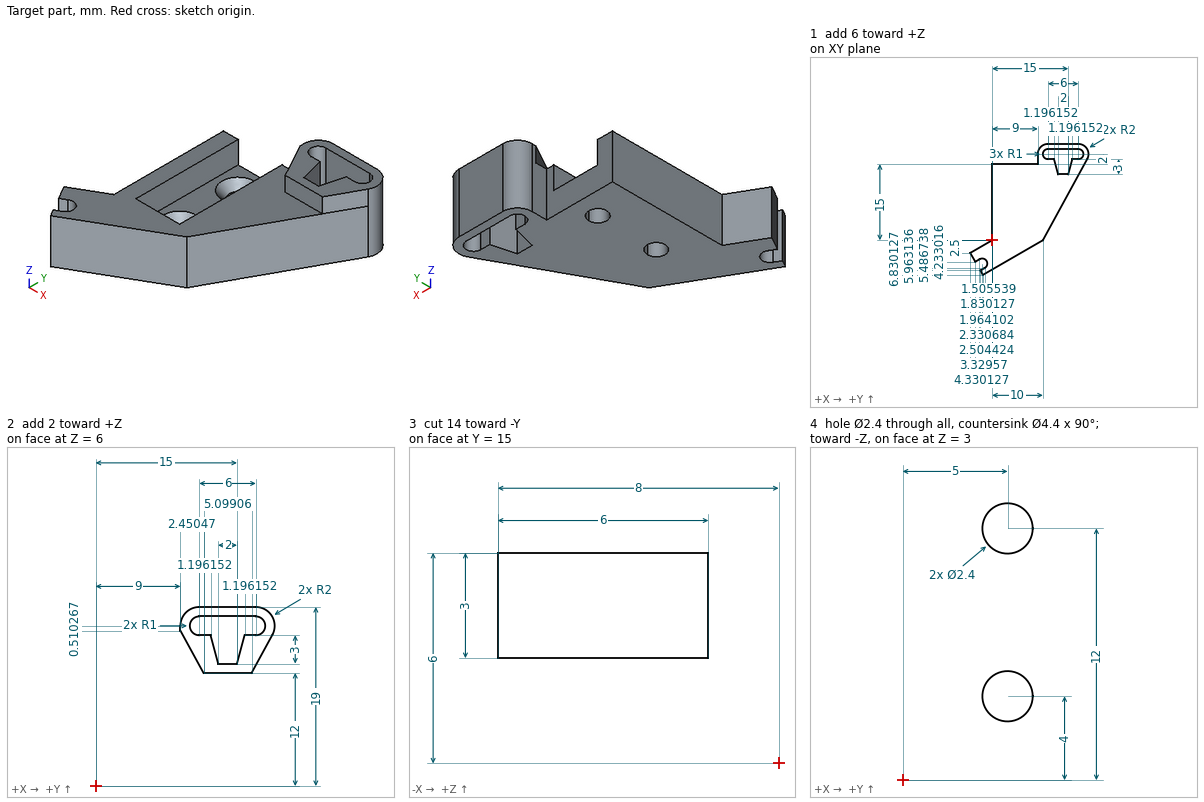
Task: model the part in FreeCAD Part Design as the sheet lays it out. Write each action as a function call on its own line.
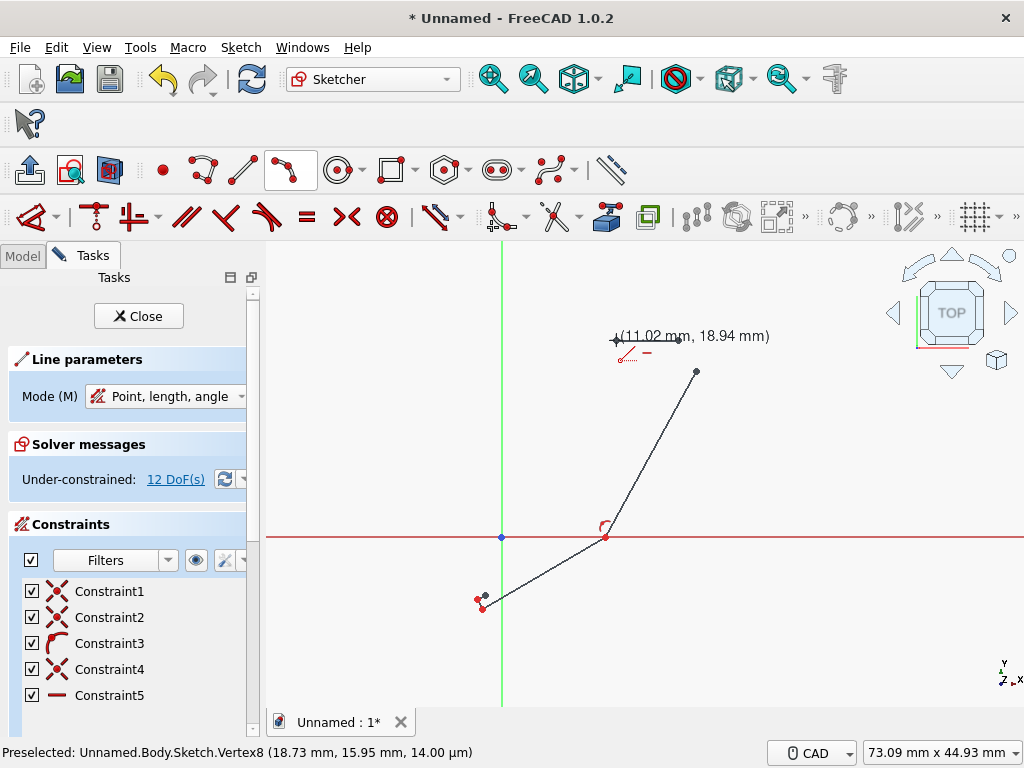
click(204, 170)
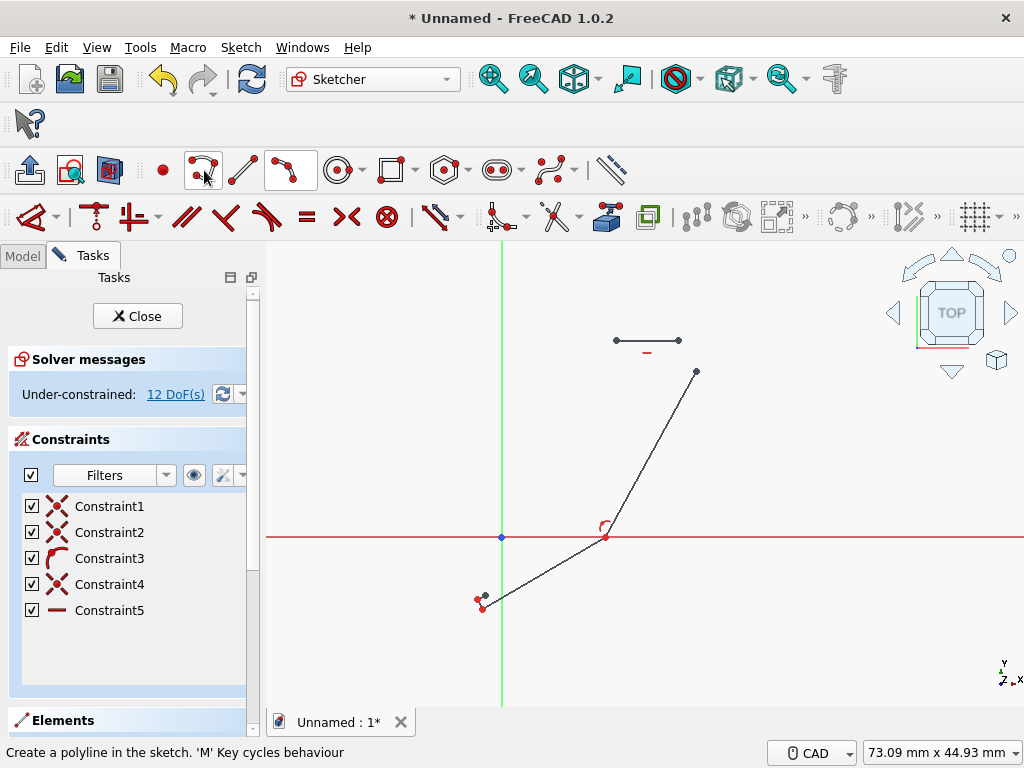
click(595, 361)
click(595, 382)
click(502, 382)
click(502, 537)
click(457, 563)
click(467, 581)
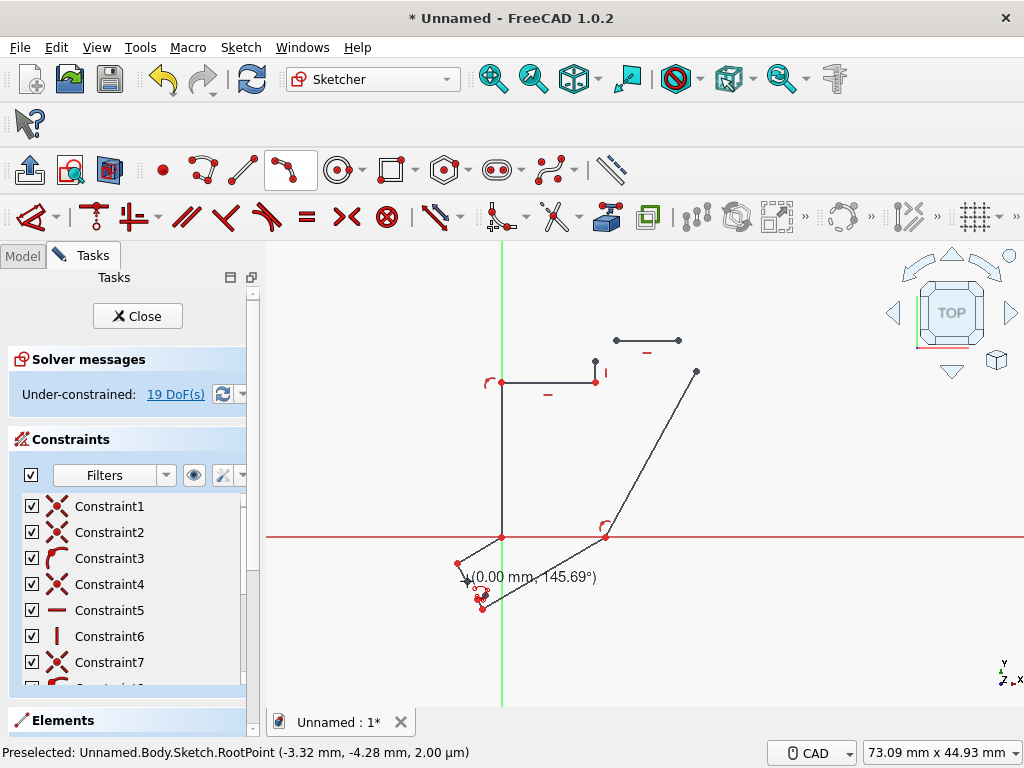
scroll(476, 576, up, 3)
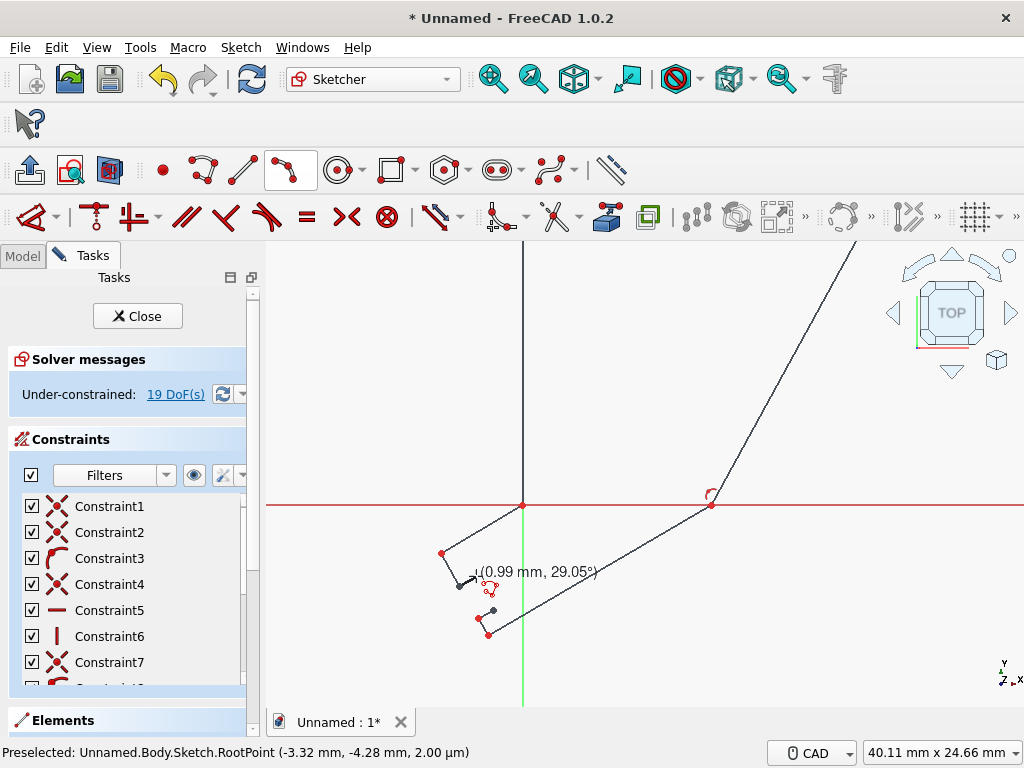
click(475, 576)
right_click(475, 576)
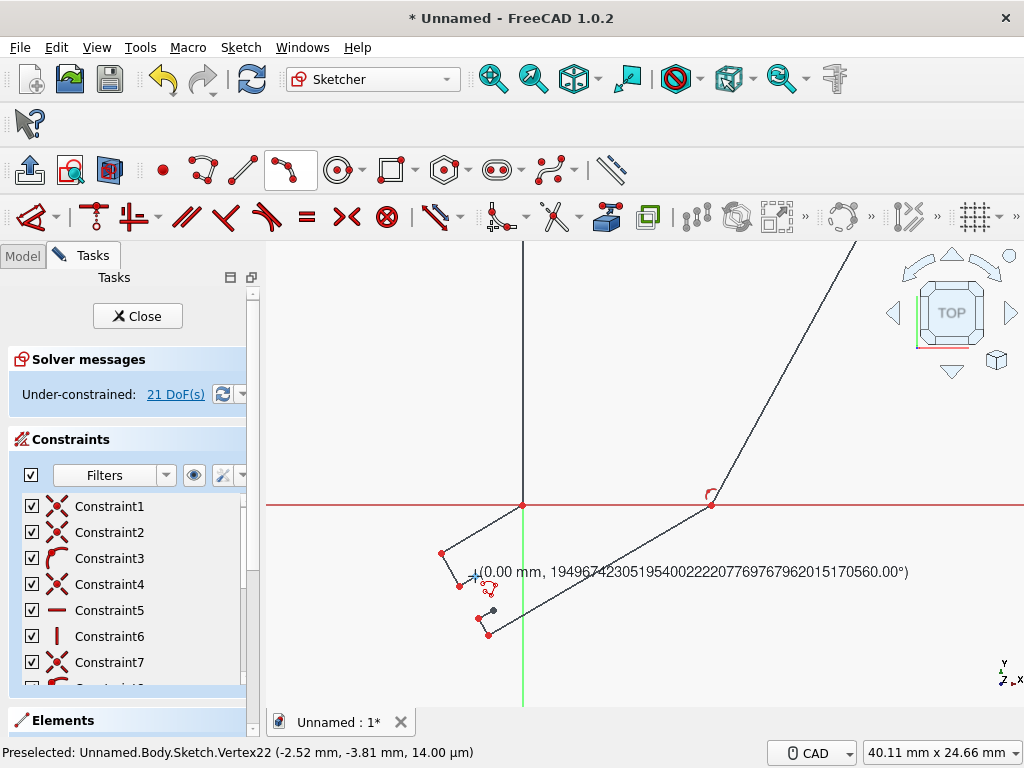
key(g)
key(3)
key(a)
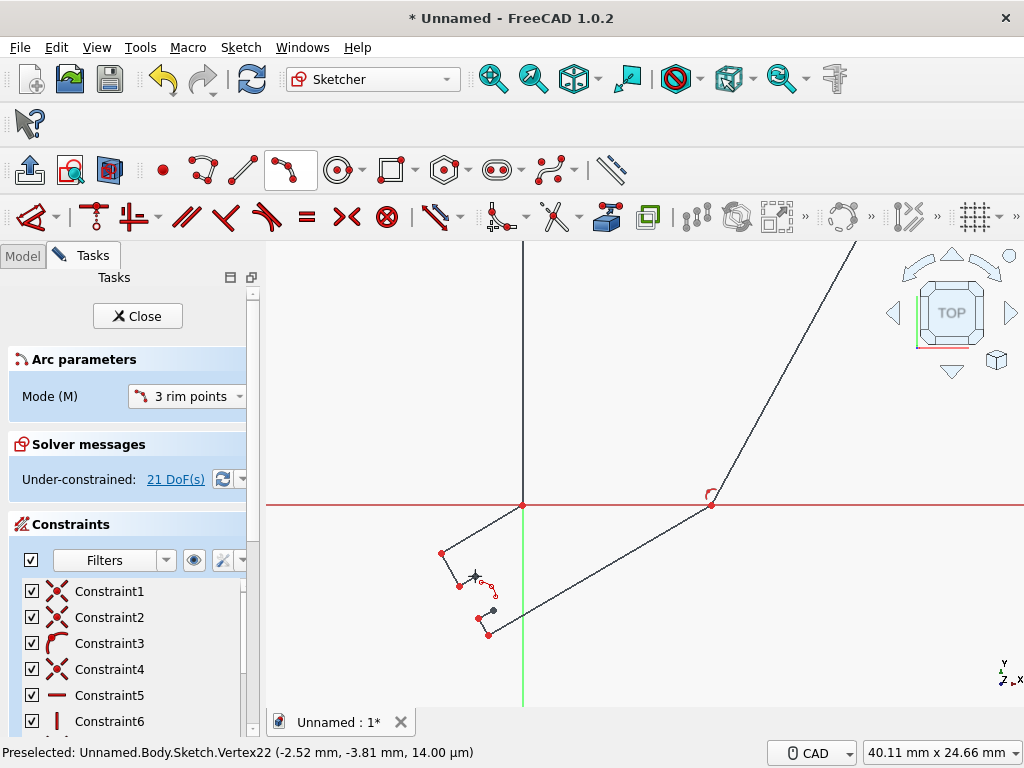
scroll(476, 576, down, 3)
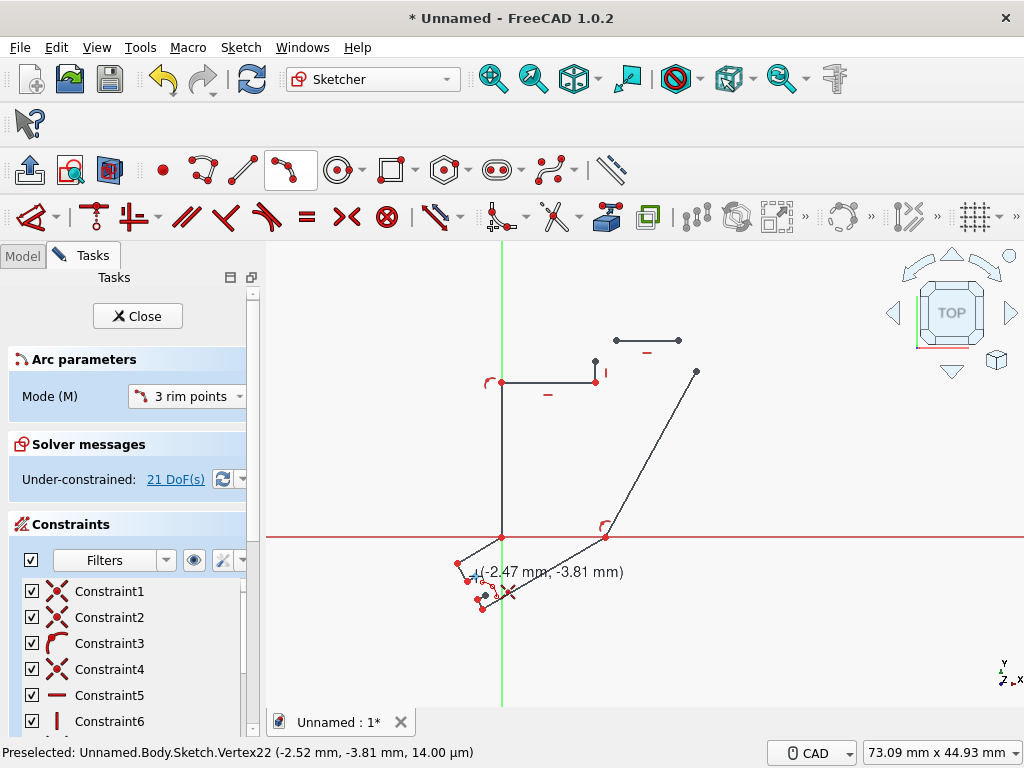
click(696, 372)
click(678, 341)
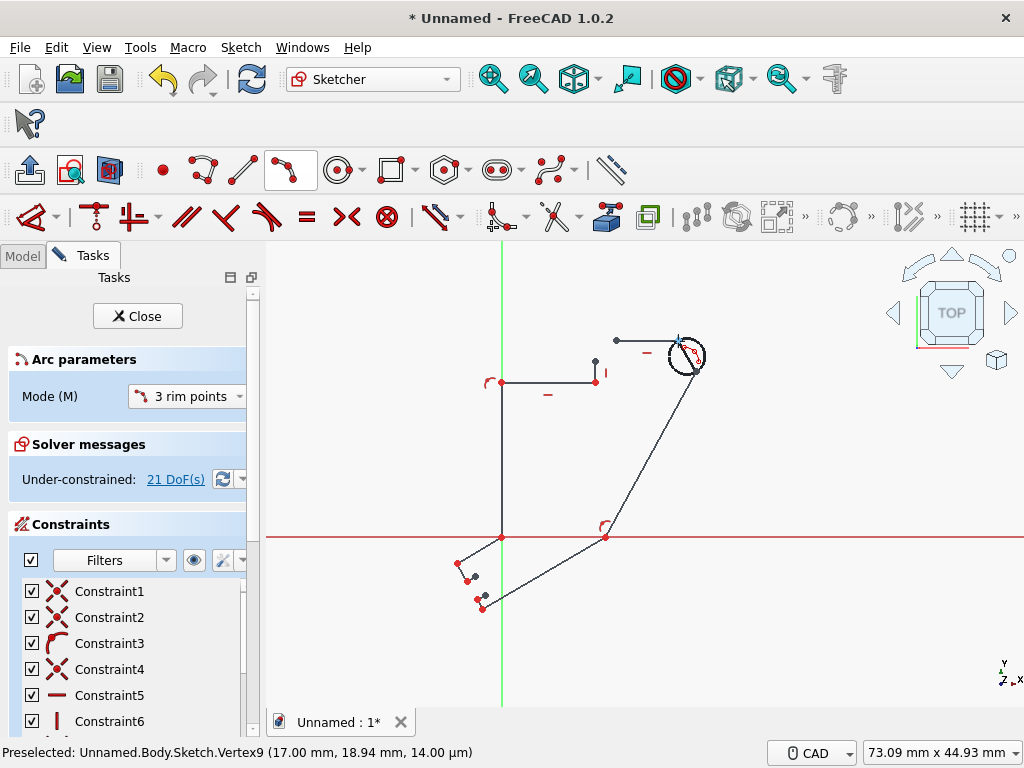
scroll(696, 350, up, 3)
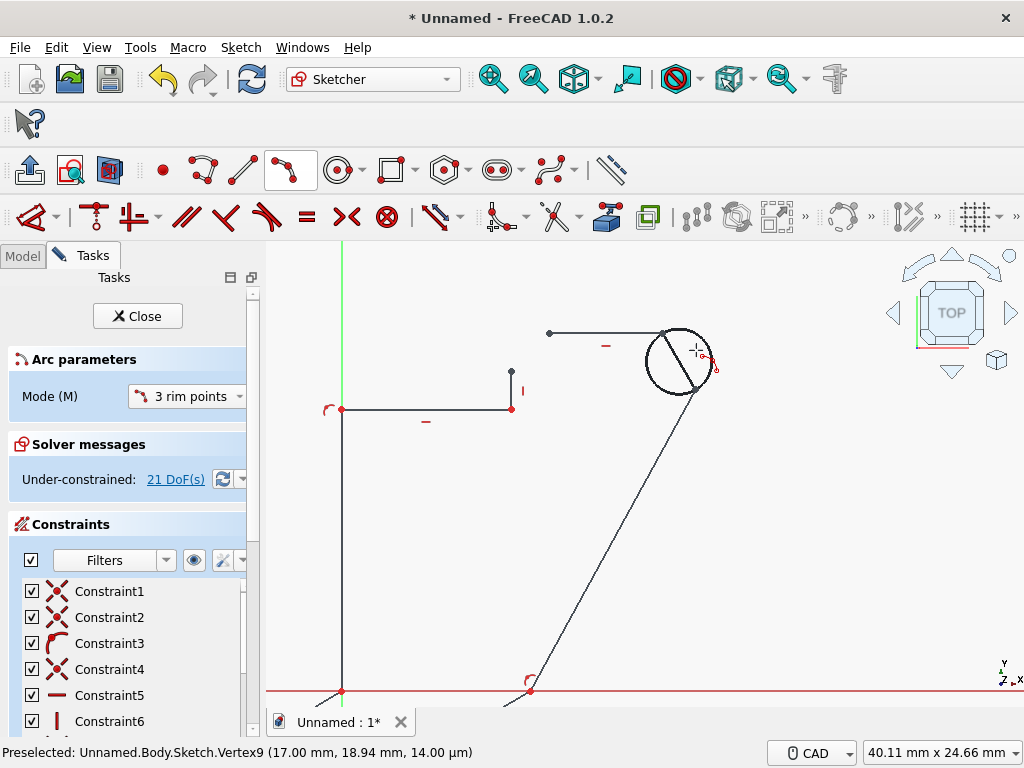
click(695, 351)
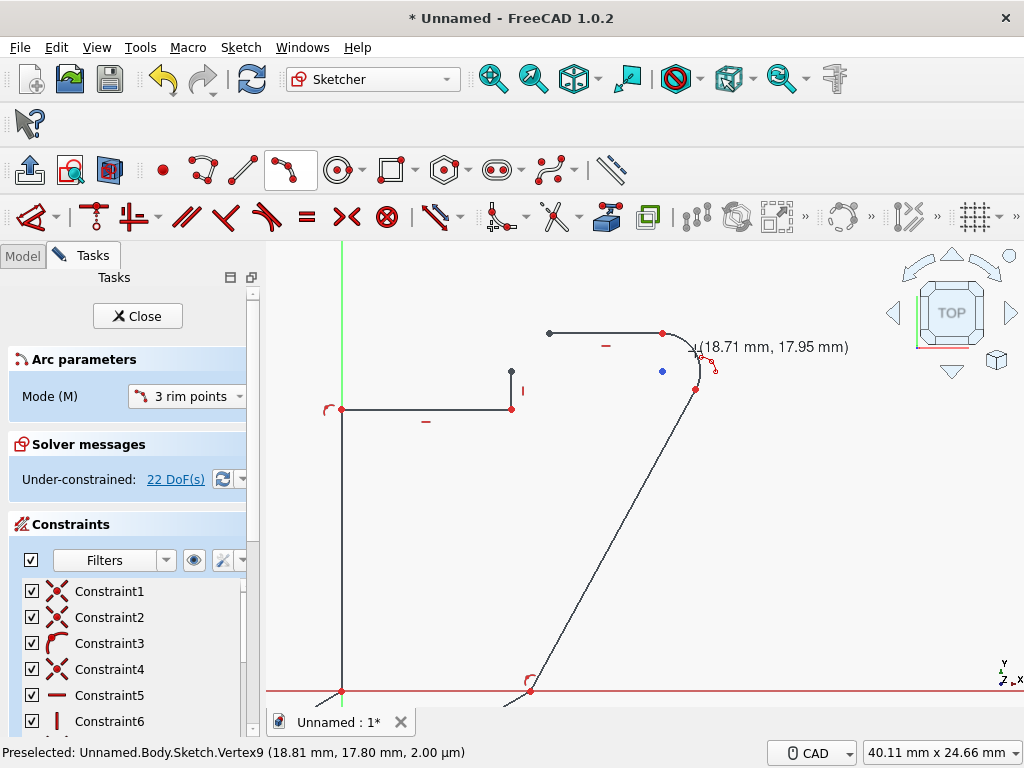
click(550, 333)
click(511, 372)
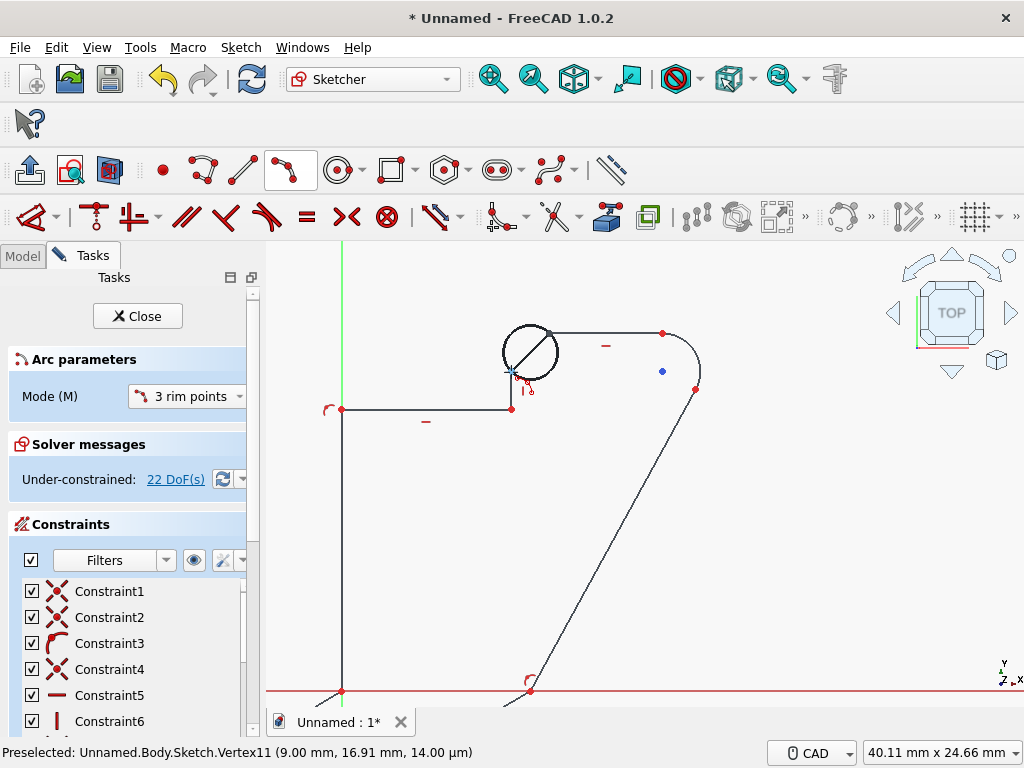
scroll(523, 343, up, 2)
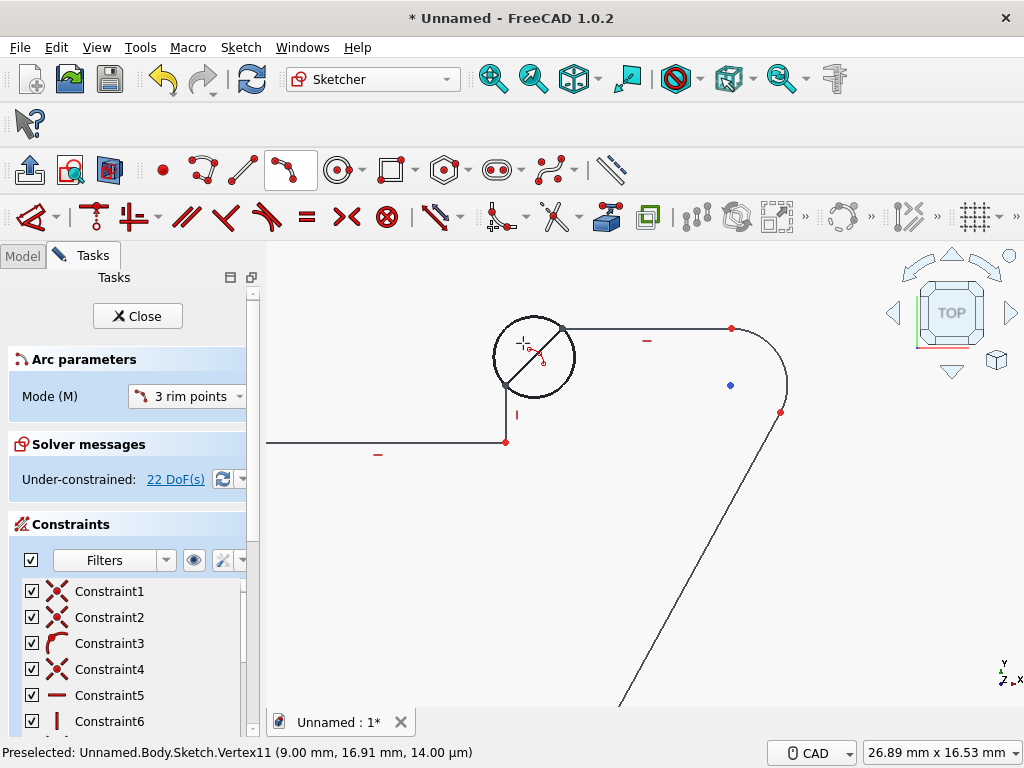
click(522, 343)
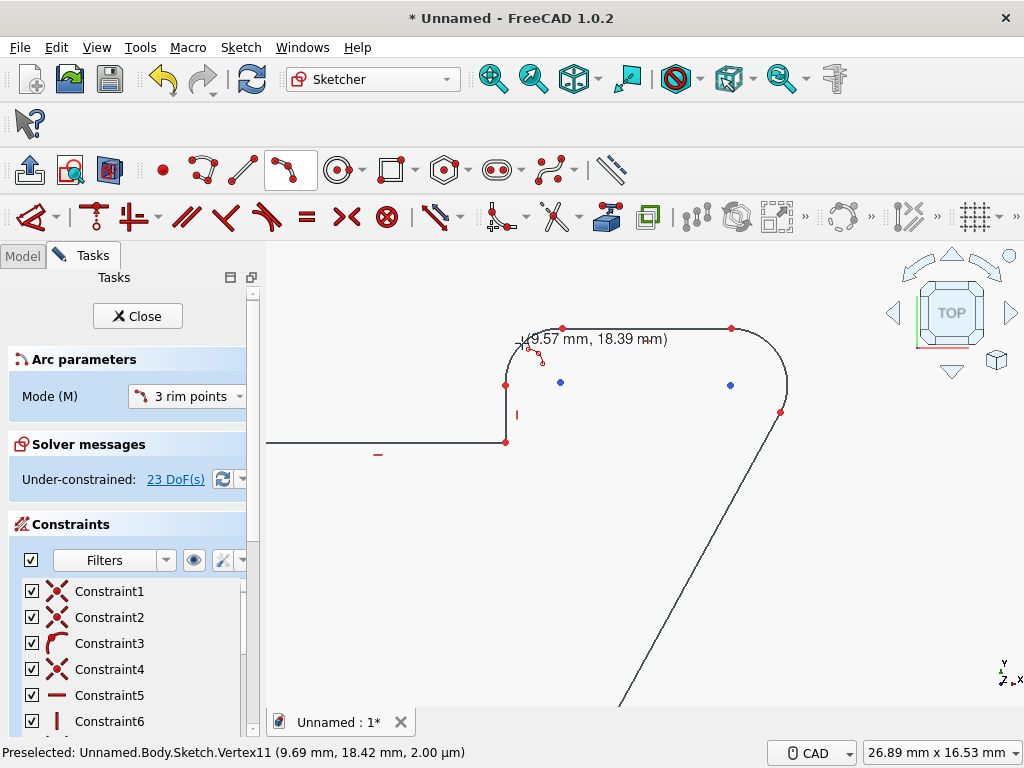
scroll(647, 348, down, 5)